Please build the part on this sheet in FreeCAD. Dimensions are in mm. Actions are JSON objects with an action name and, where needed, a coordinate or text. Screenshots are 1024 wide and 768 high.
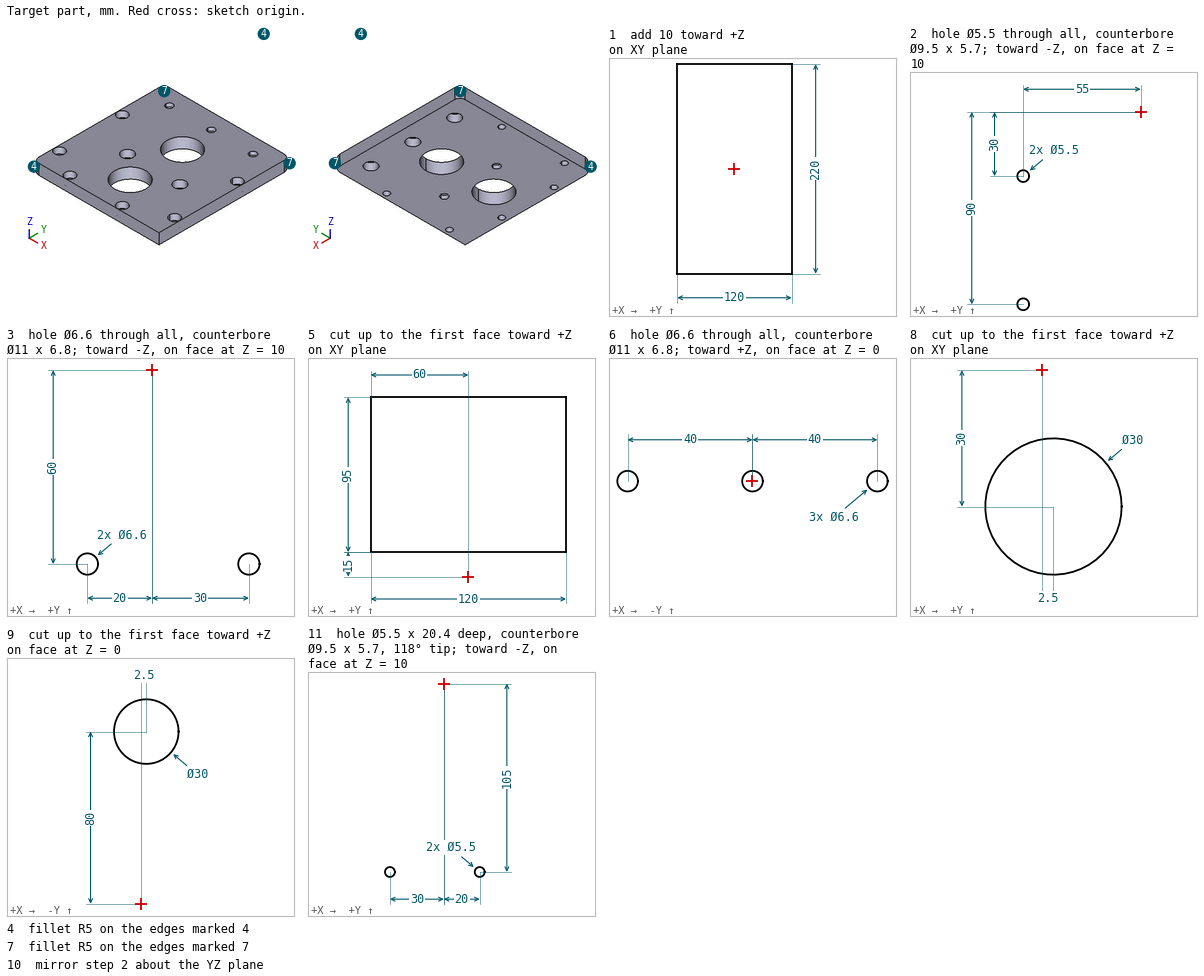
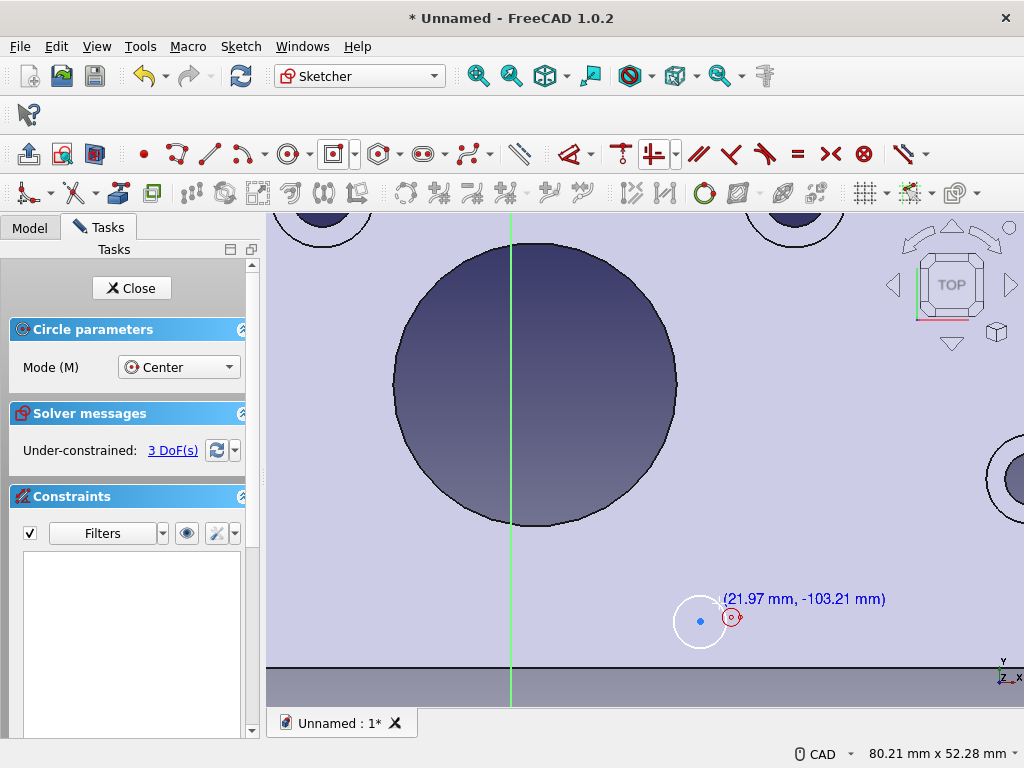
{"action": "scroll", "coordinate": [625, 599], "scroll_direction": "down", "scroll_amount": 6}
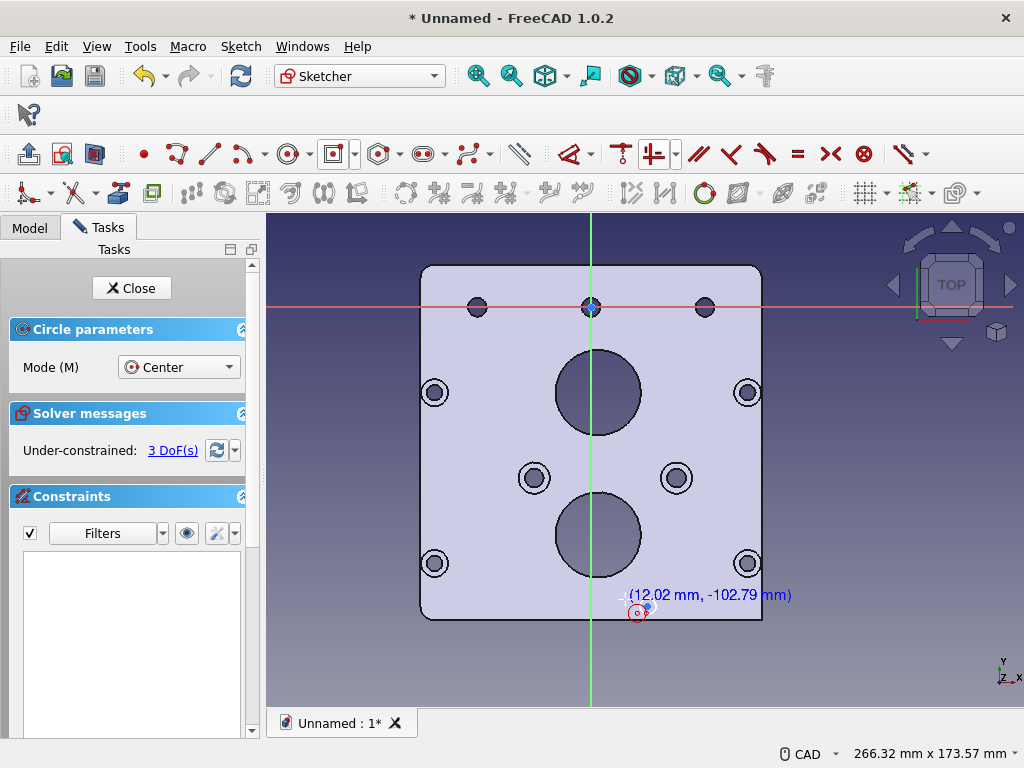
{"action": "scroll", "coordinate": [506, 606], "scroll_direction": "up", "scroll_amount": 6}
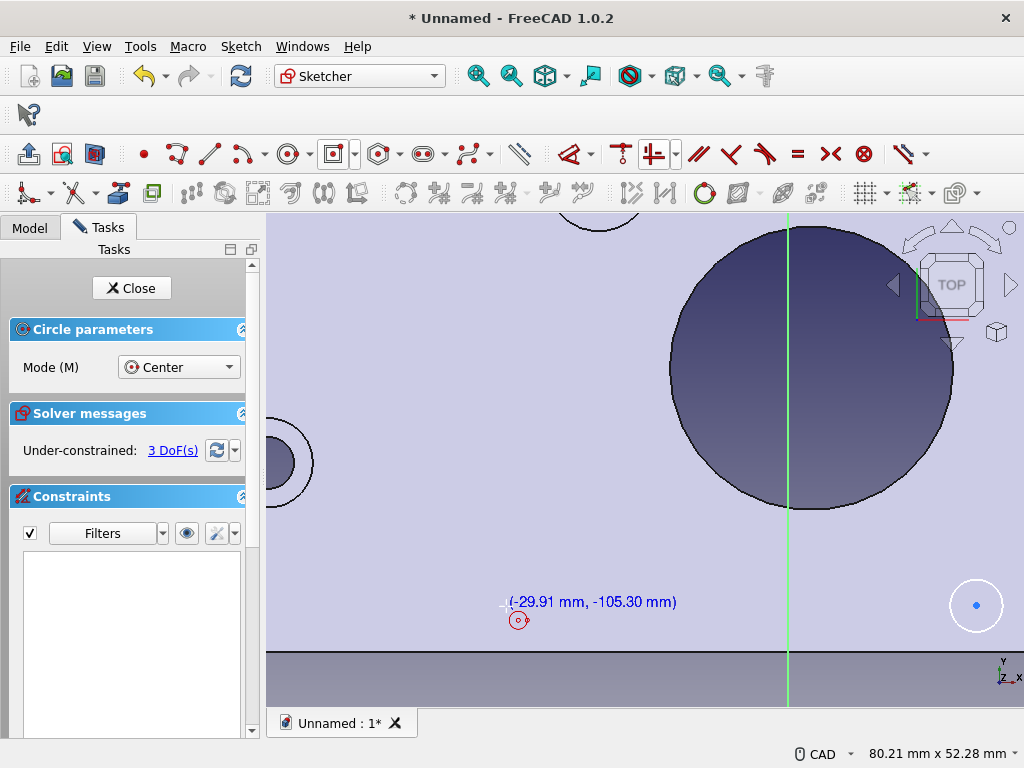
{"action": "left_click", "coordinate": [504, 605]}
{"action": "left_click", "coordinate": [523, 586]}
{"action": "key", "text": "Escape"}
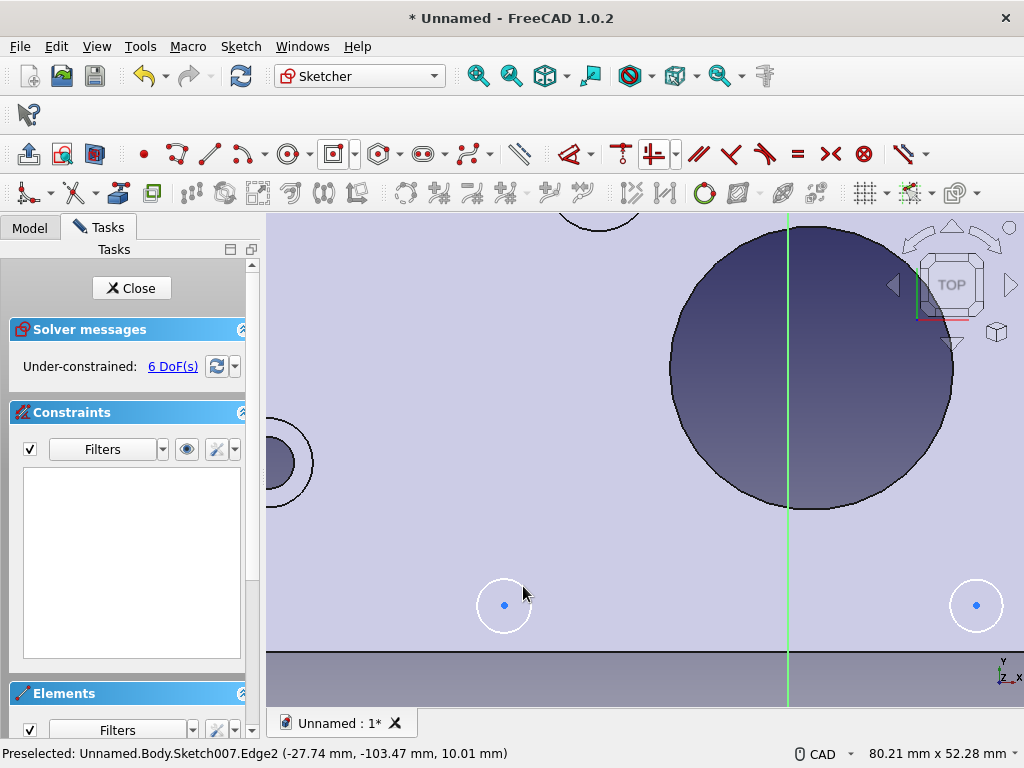
{"action": "scroll", "coordinate": [506, 606], "scroll_direction": "down", "scroll_amount": 6}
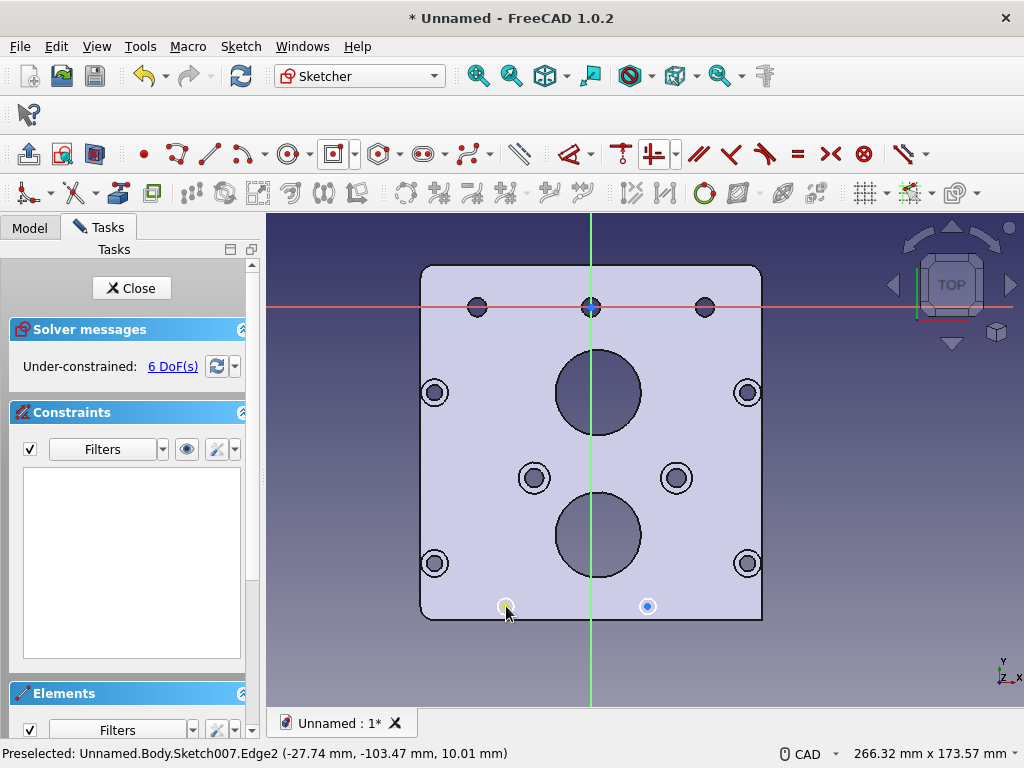
{"action": "scroll", "coordinate": [653, 601], "scroll_direction": "up", "scroll_amount": 3}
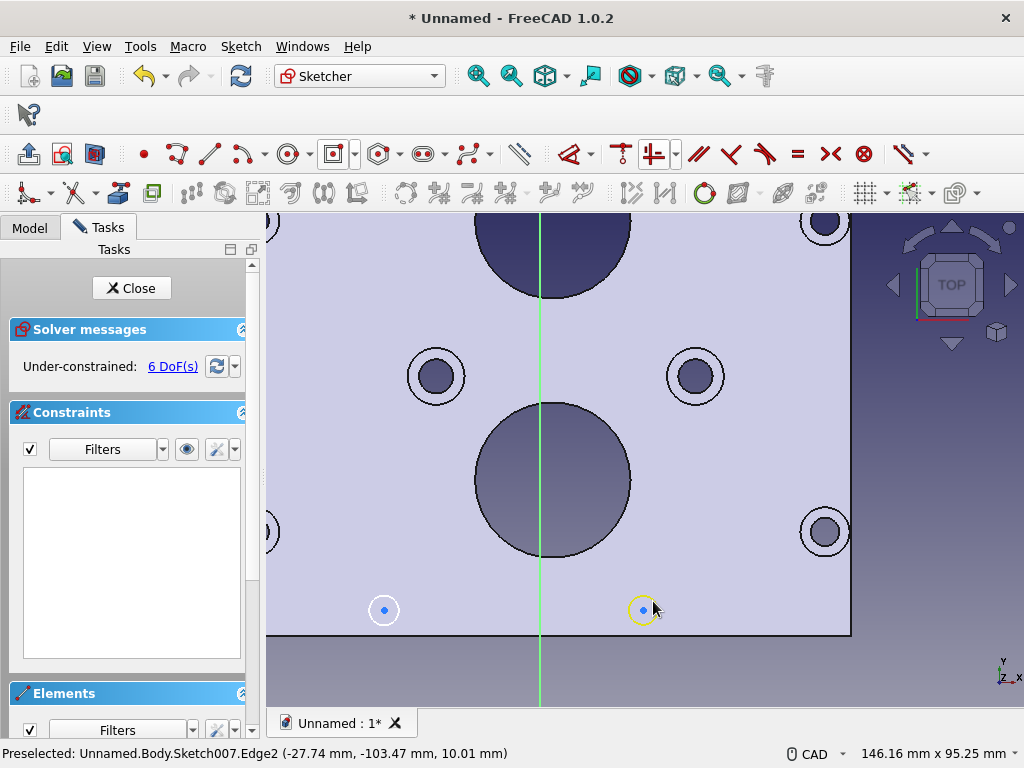
{"action": "left_click", "coordinate": [653, 600]}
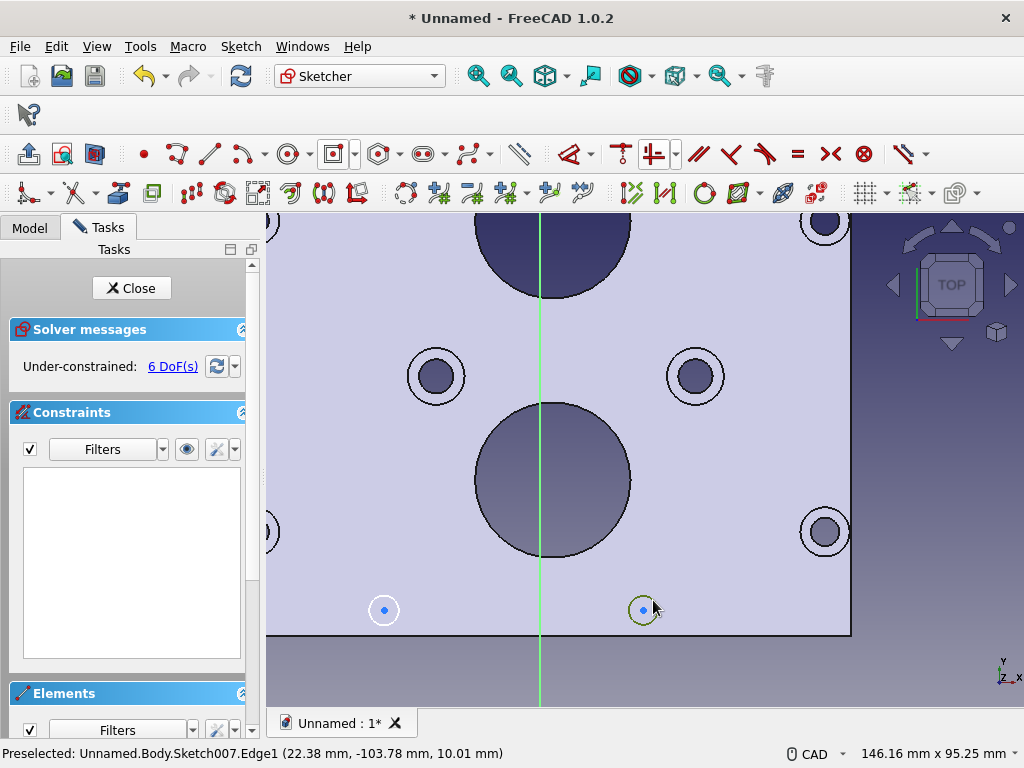
{"action": "left_click", "coordinate": [394, 600]}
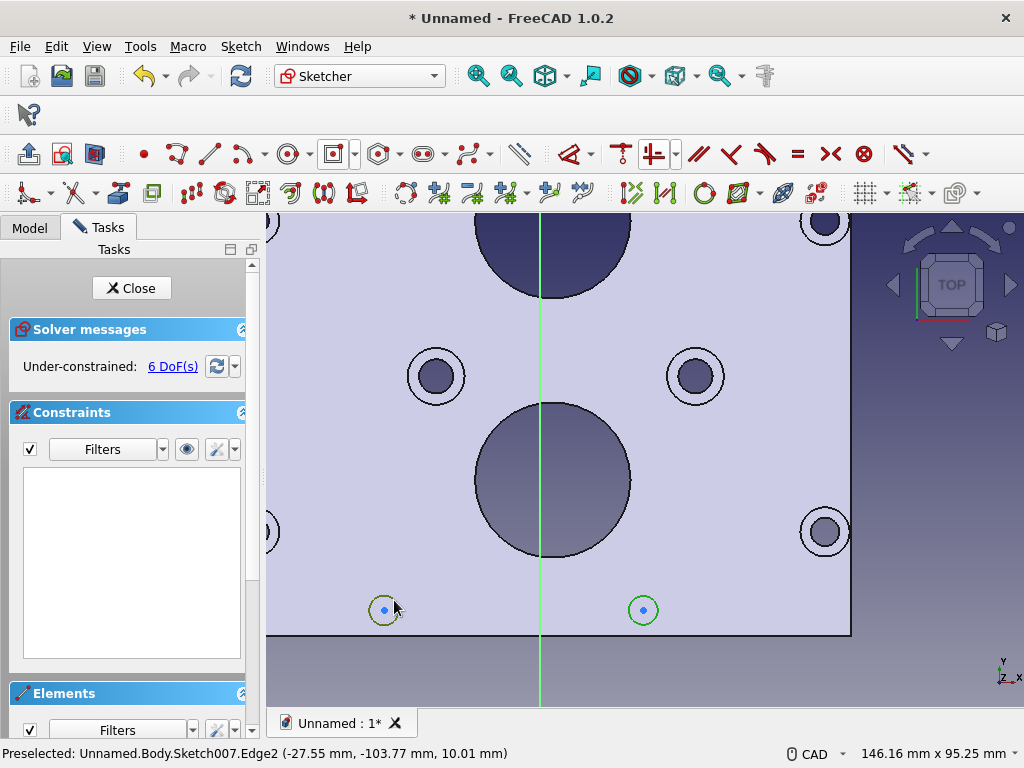
{"action": "left_click", "coordinate": [798, 154]}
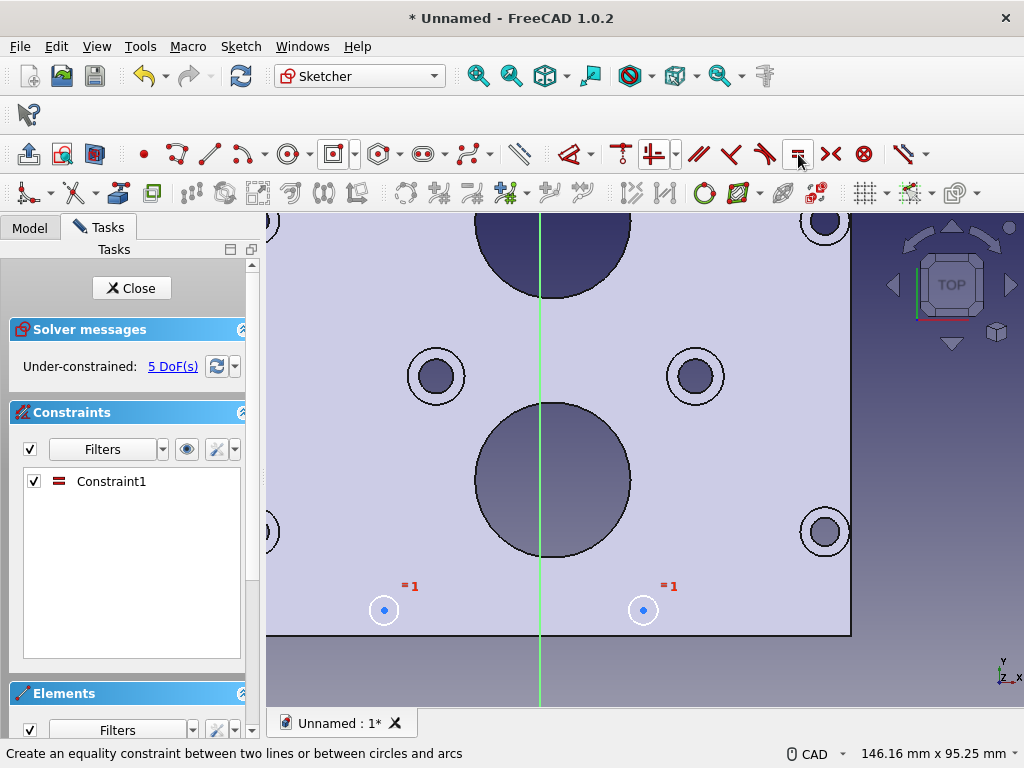
{"action": "left_click", "coordinate": [643, 610]}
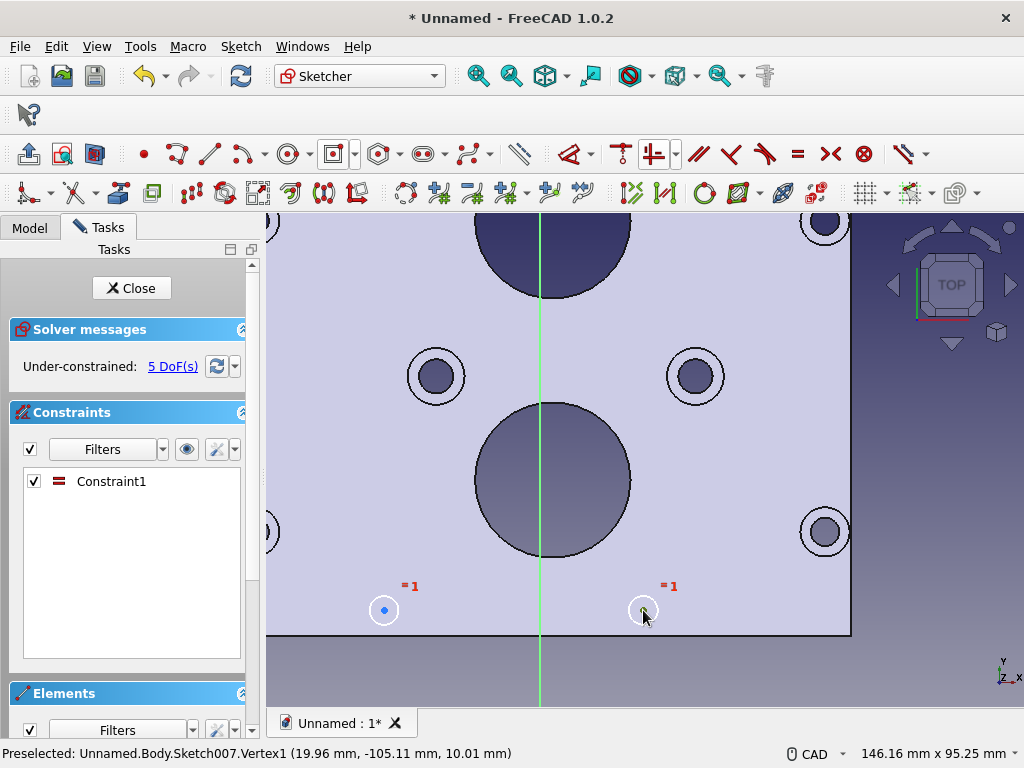
{"action": "left_click", "coordinate": [384, 610]}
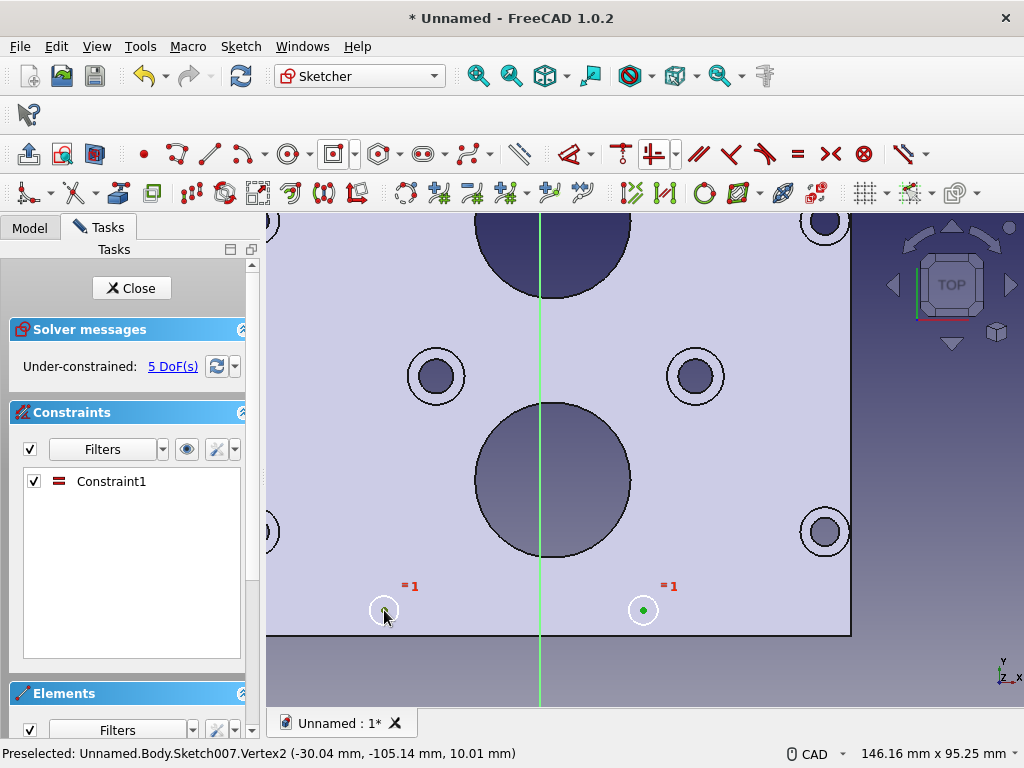
{"action": "key", "text": "h"}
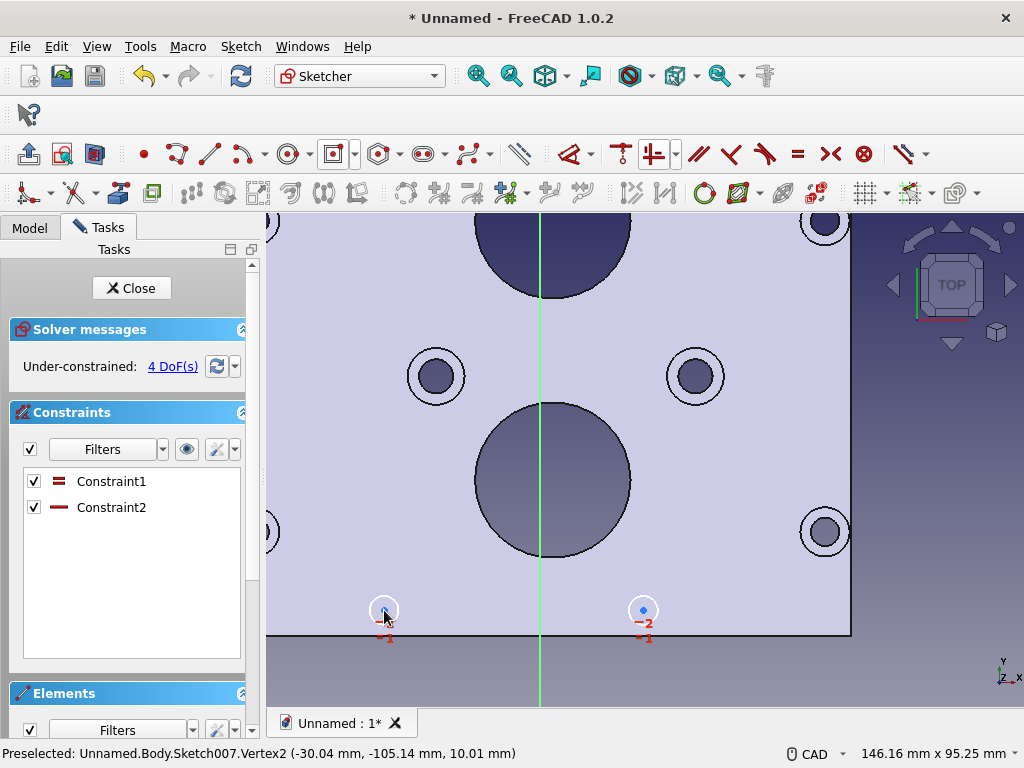
{"action": "left_click", "coordinate": [568, 154]}